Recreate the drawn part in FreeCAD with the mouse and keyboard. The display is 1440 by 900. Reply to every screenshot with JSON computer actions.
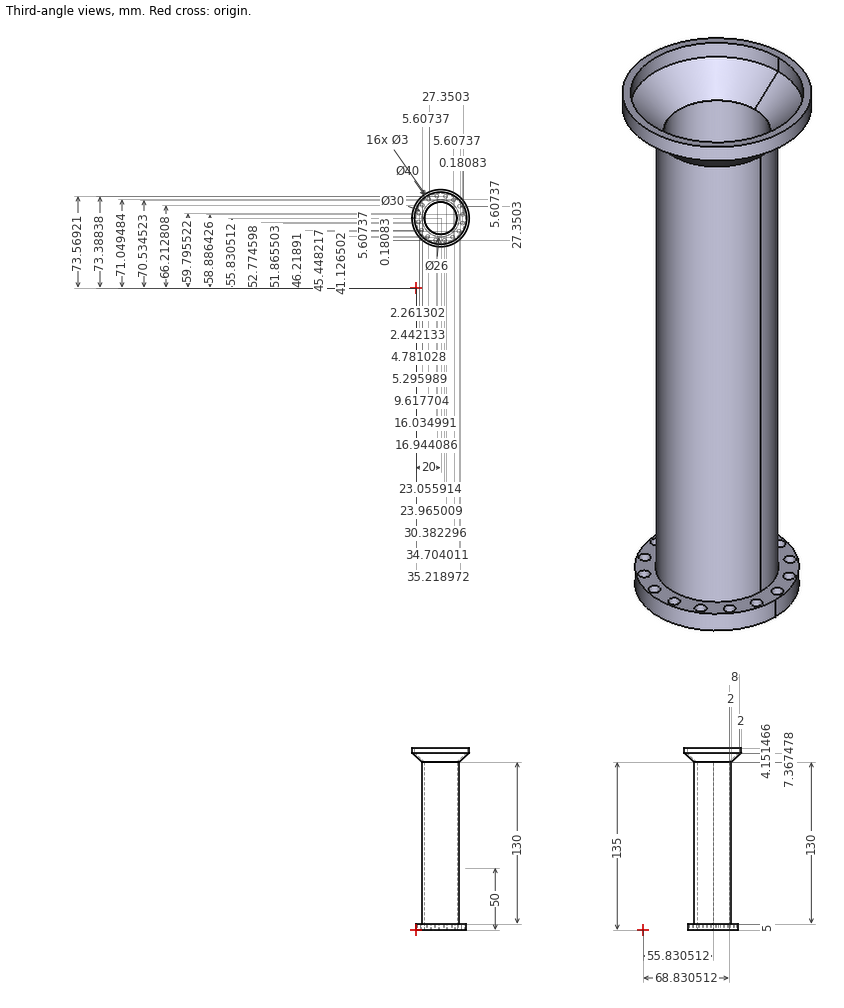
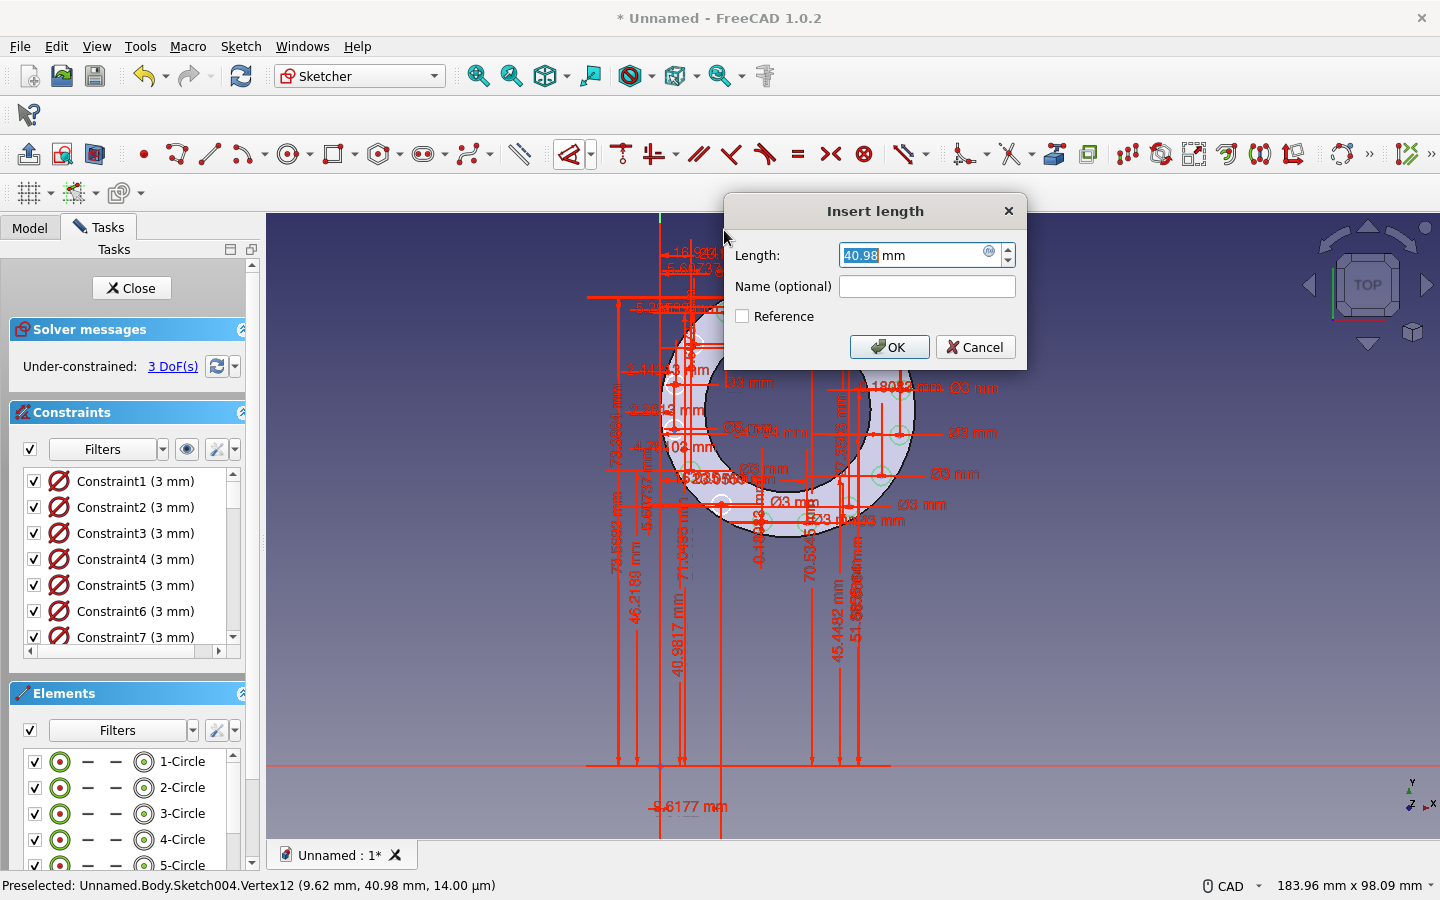
{"action": "type", "text": "41.126502"}
{"action": "key", "text": "Return"}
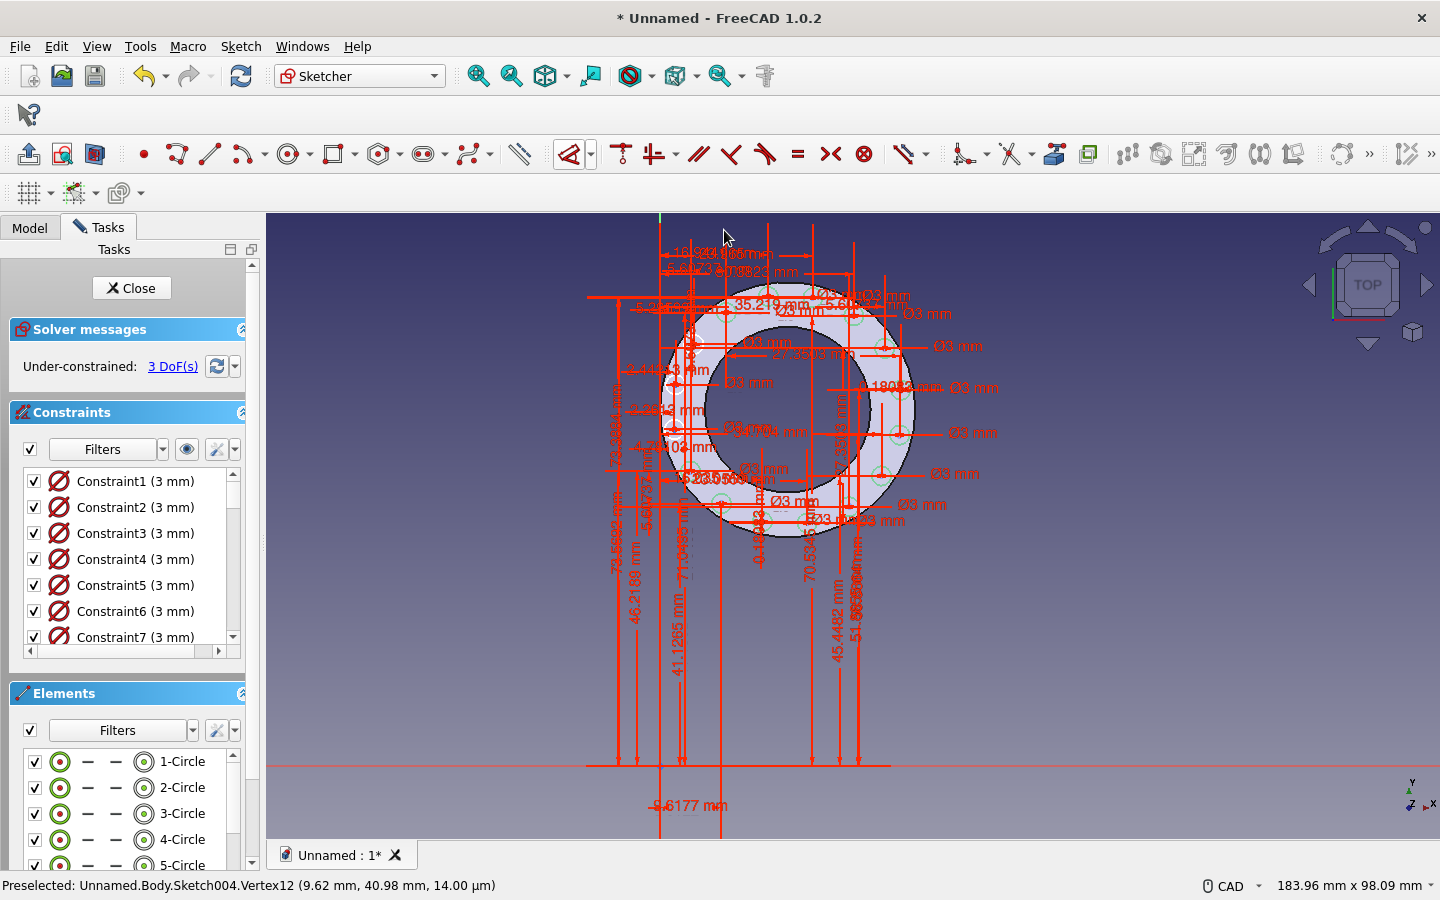
{"action": "left_click", "coordinate": [674, 429]}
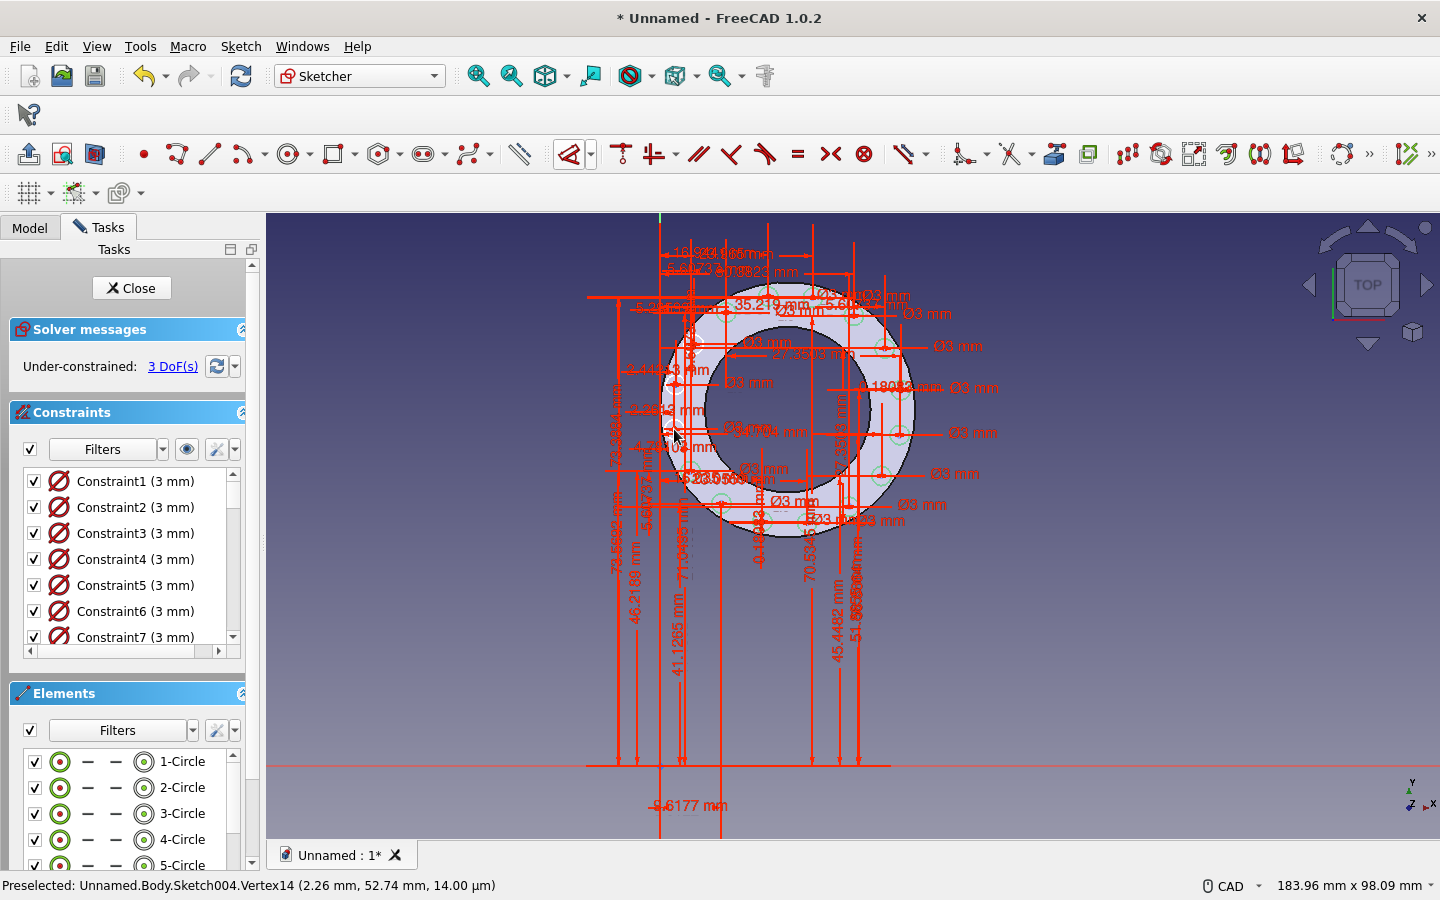
{"action": "key", "text": "i"}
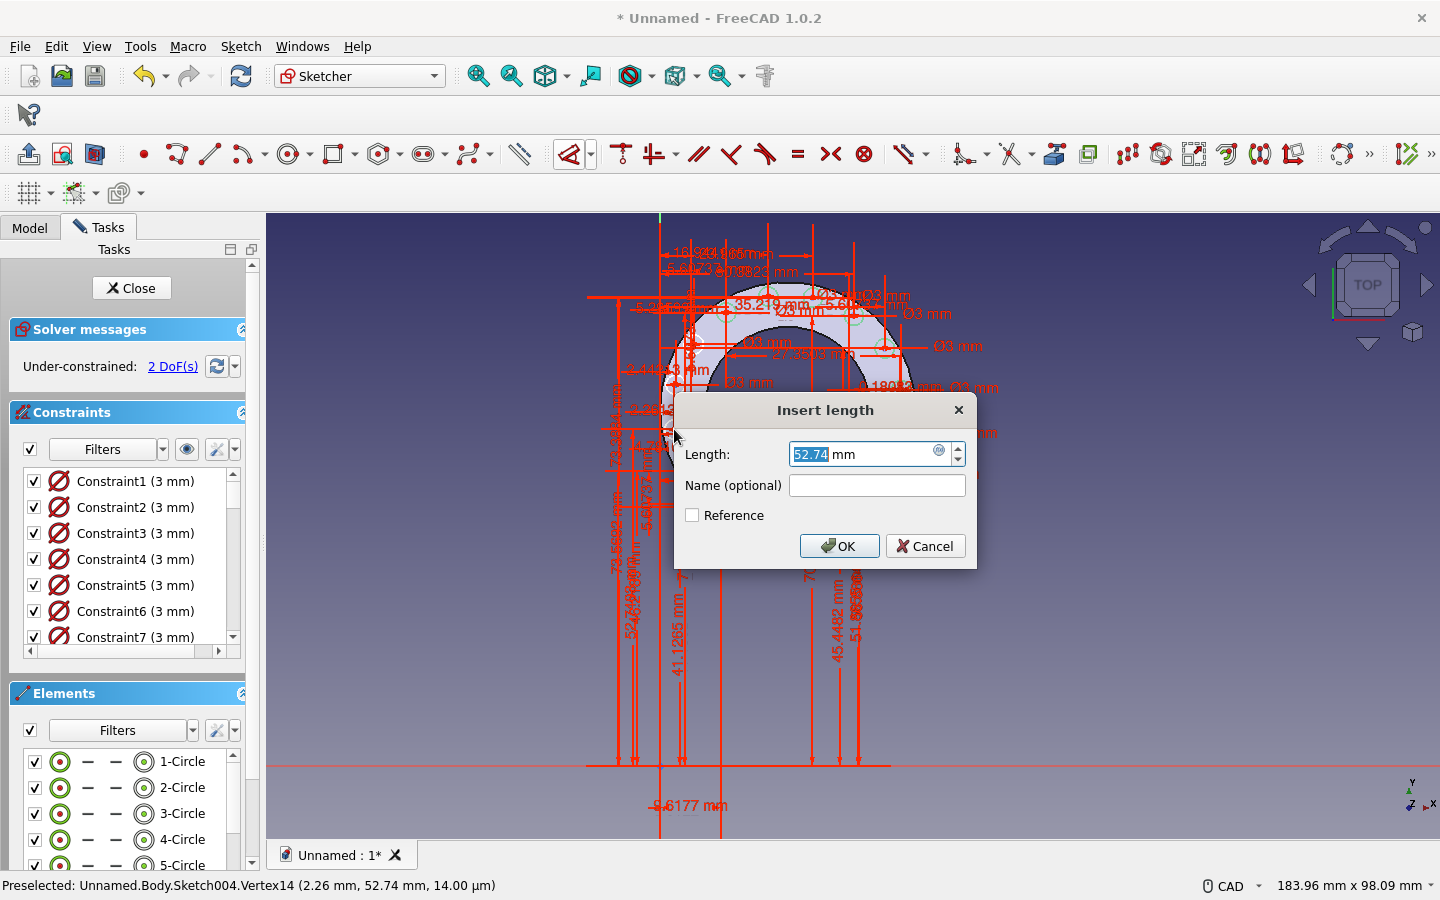
{"action": "type", "text": "52.774598"}
{"action": "key", "text": "Return"}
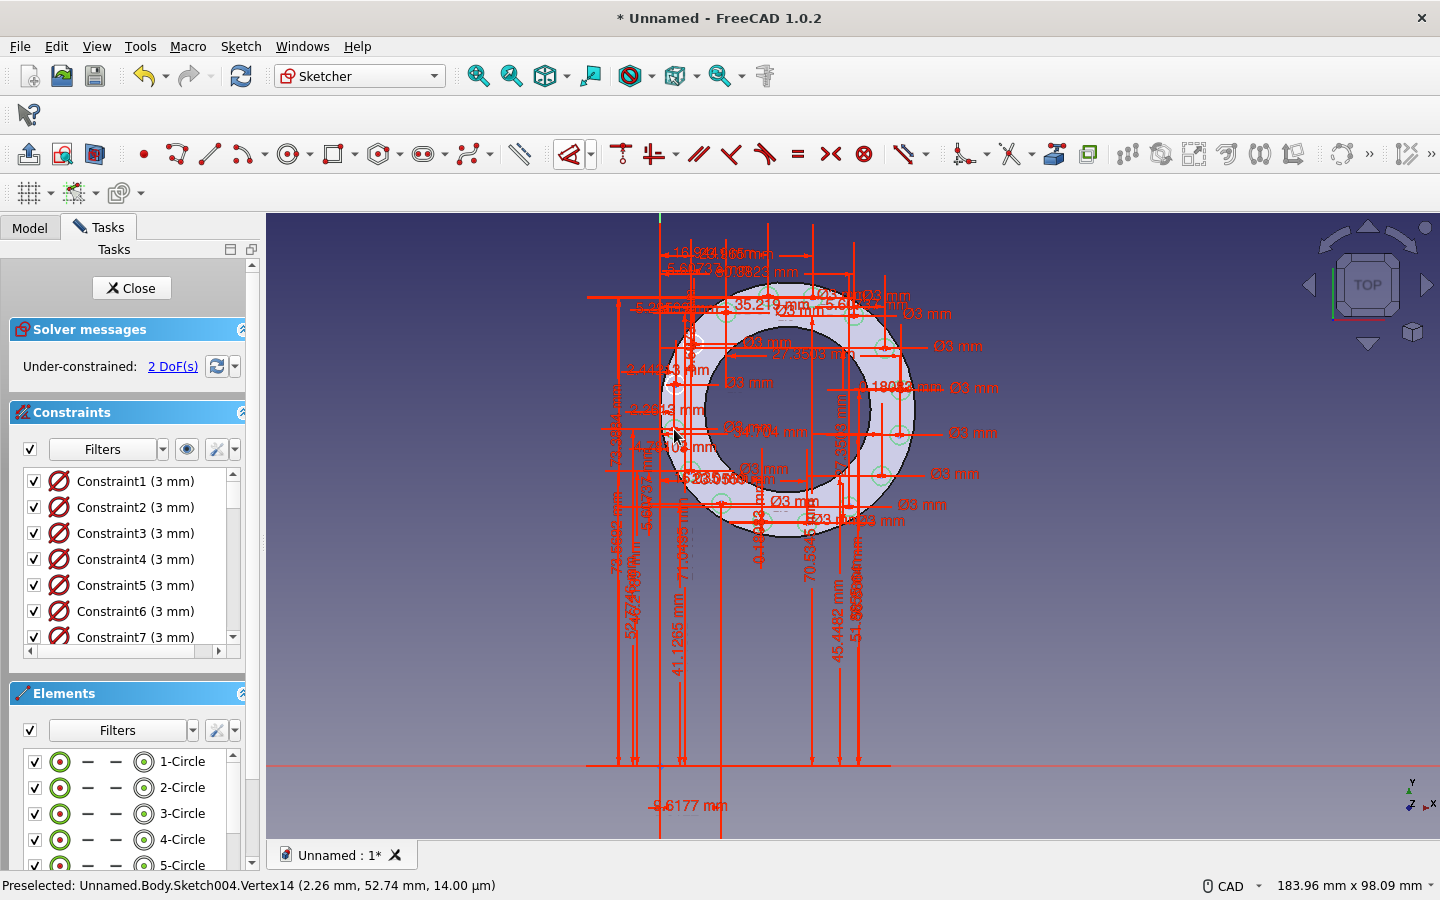
{"action": "left_click", "coordinate": [676, 385]}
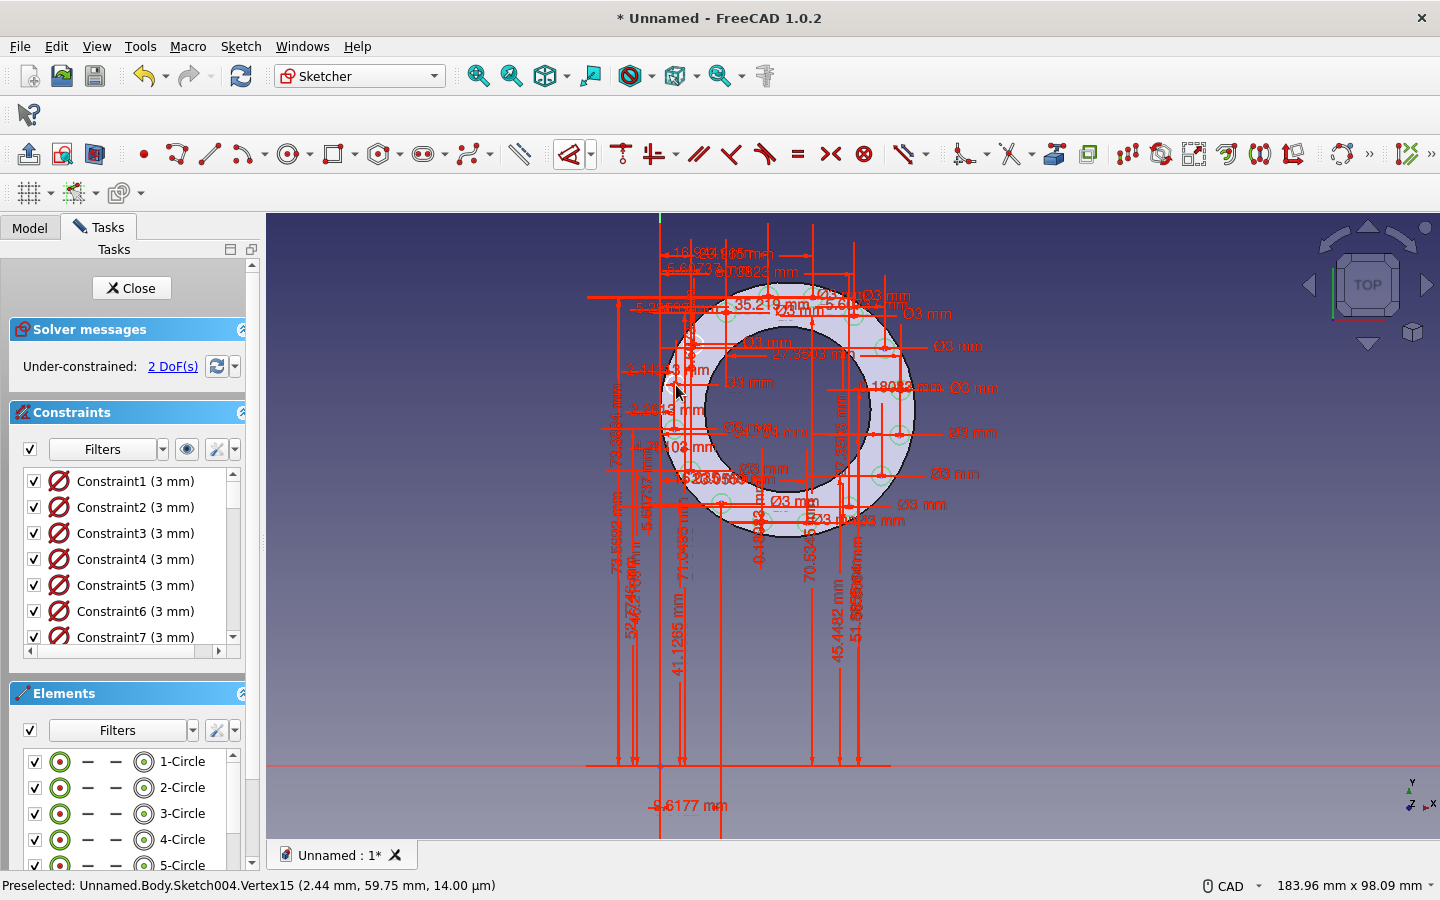
{"action": "left_click", "coordinate": [590, 154]}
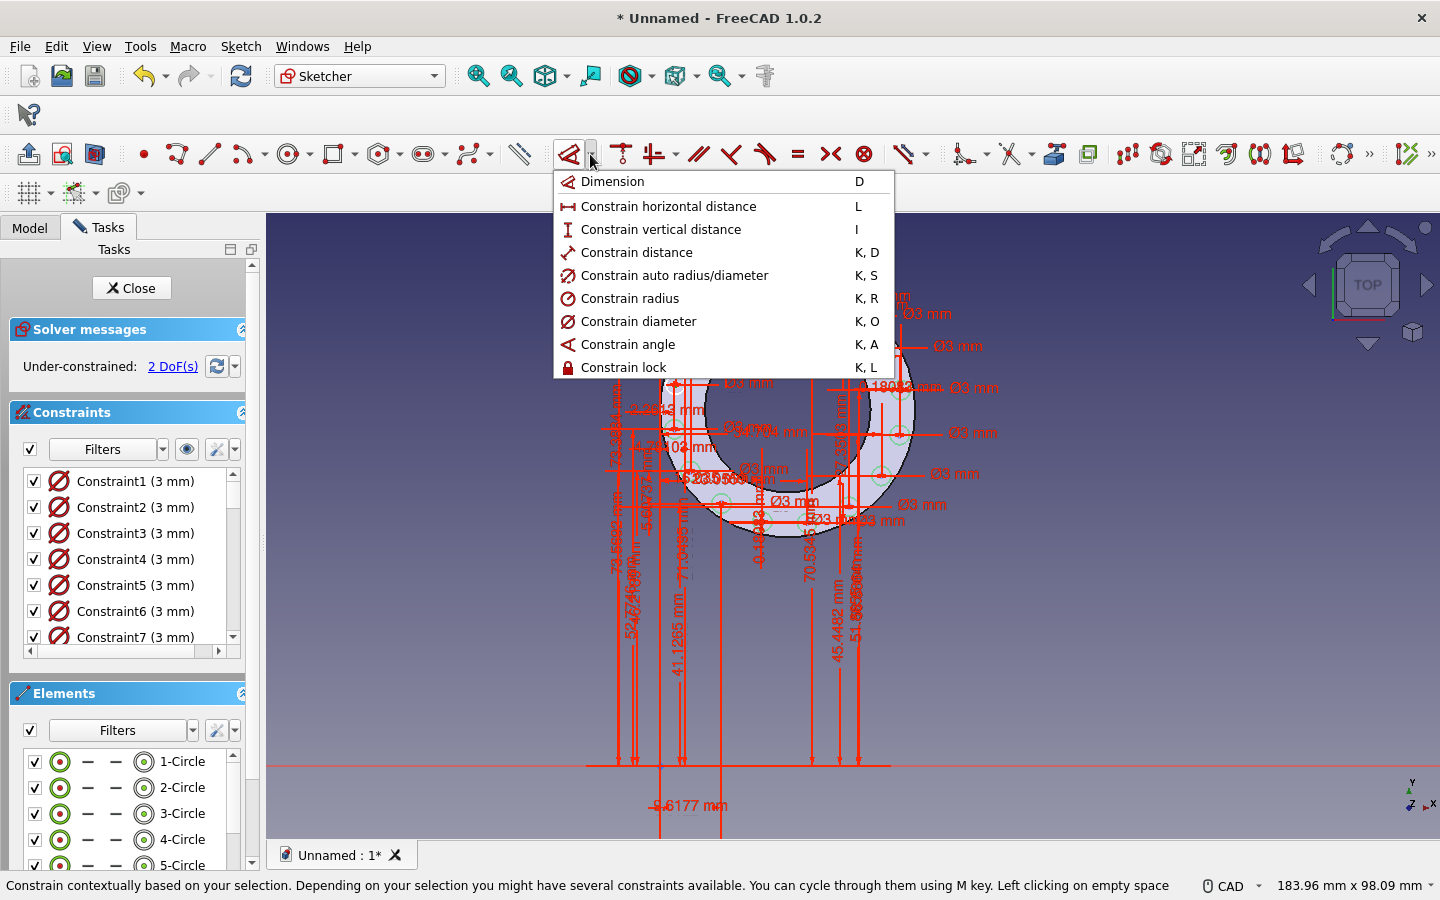
{"action": "left_click", "coordinate": [724, 230]}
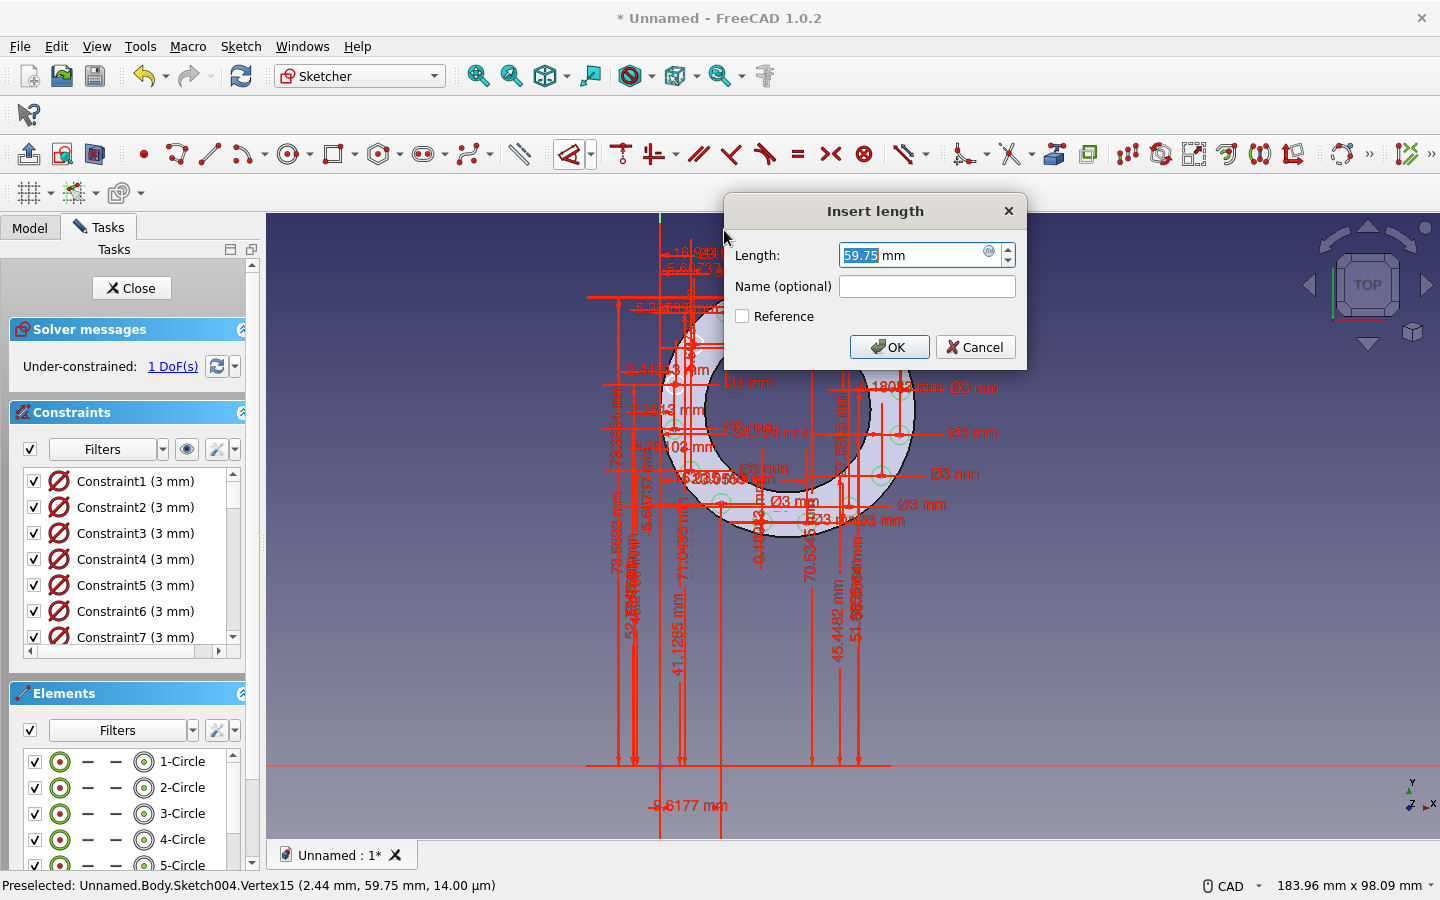
{"action": "type", "text": "59.795522"}
{"action": "key", "text": "Return"}